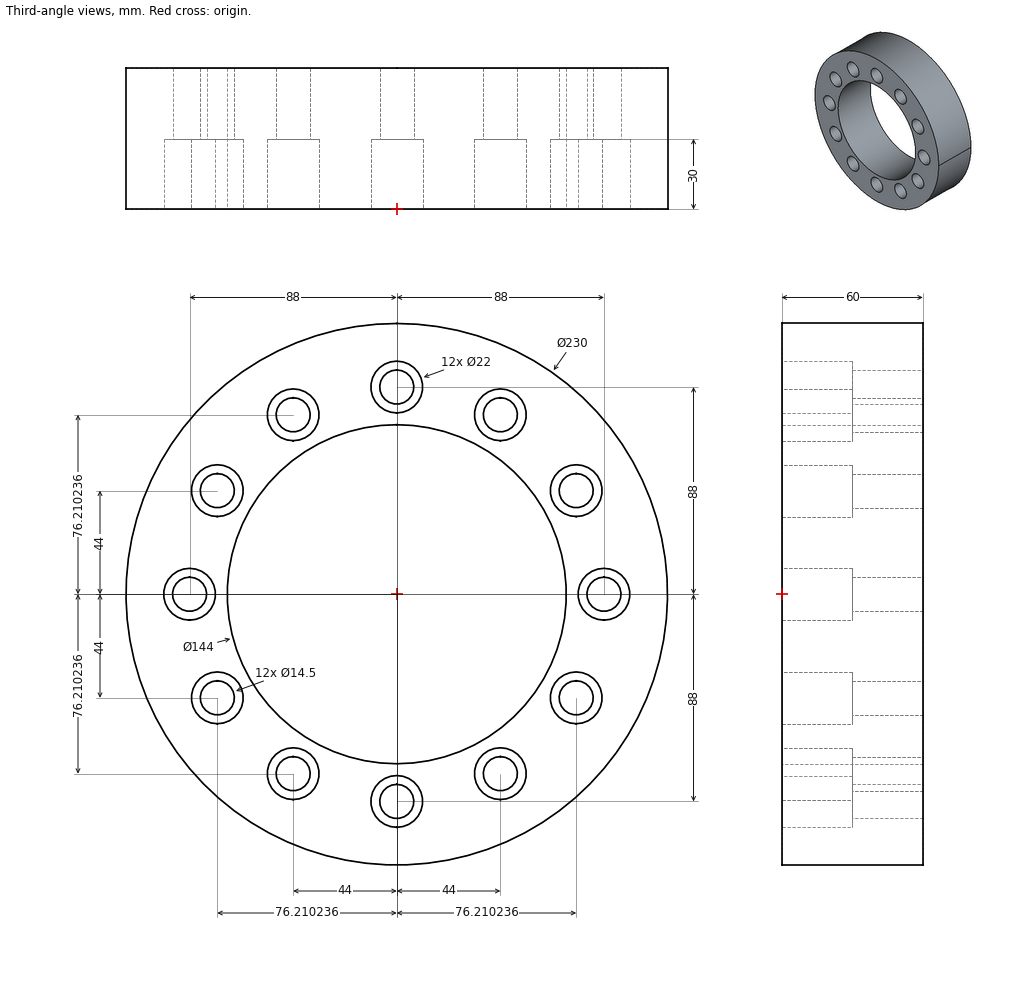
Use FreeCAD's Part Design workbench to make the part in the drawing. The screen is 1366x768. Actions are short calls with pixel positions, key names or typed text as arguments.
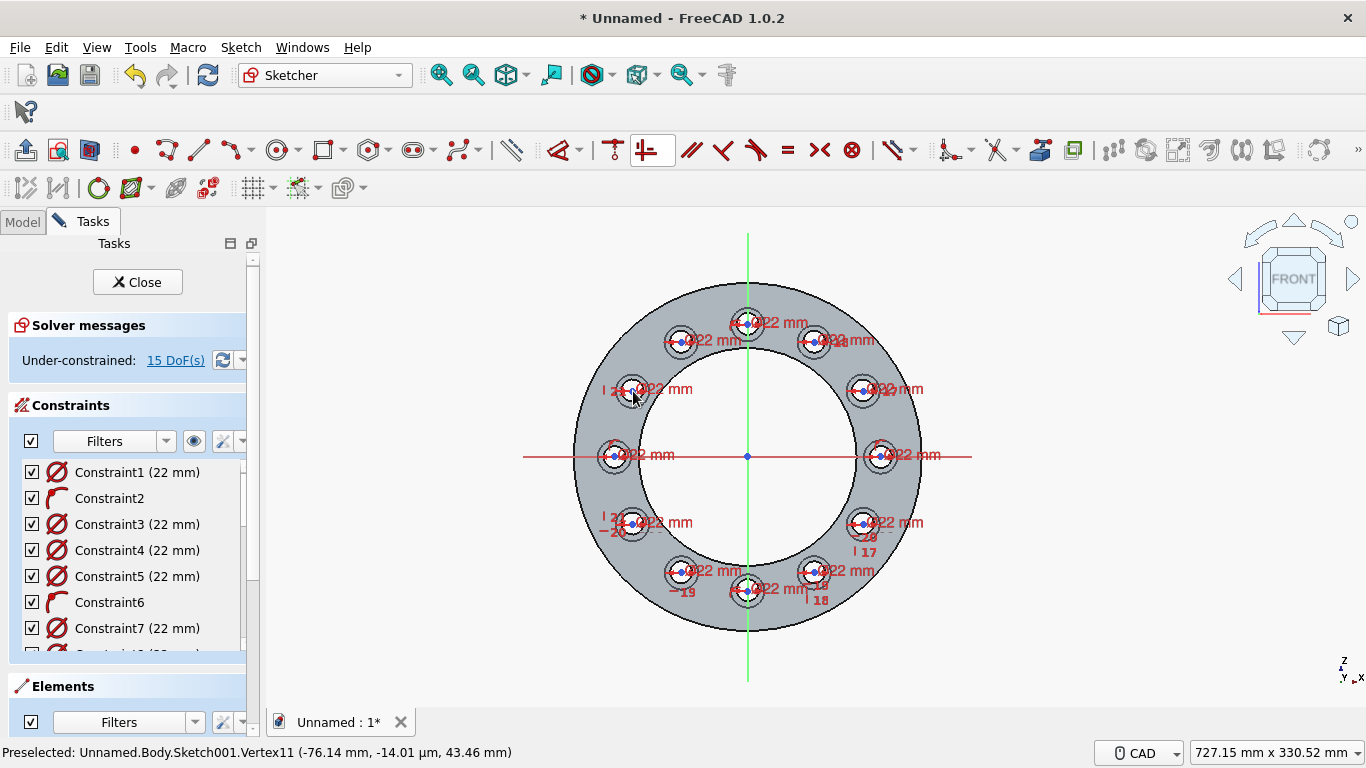
click(863, 391)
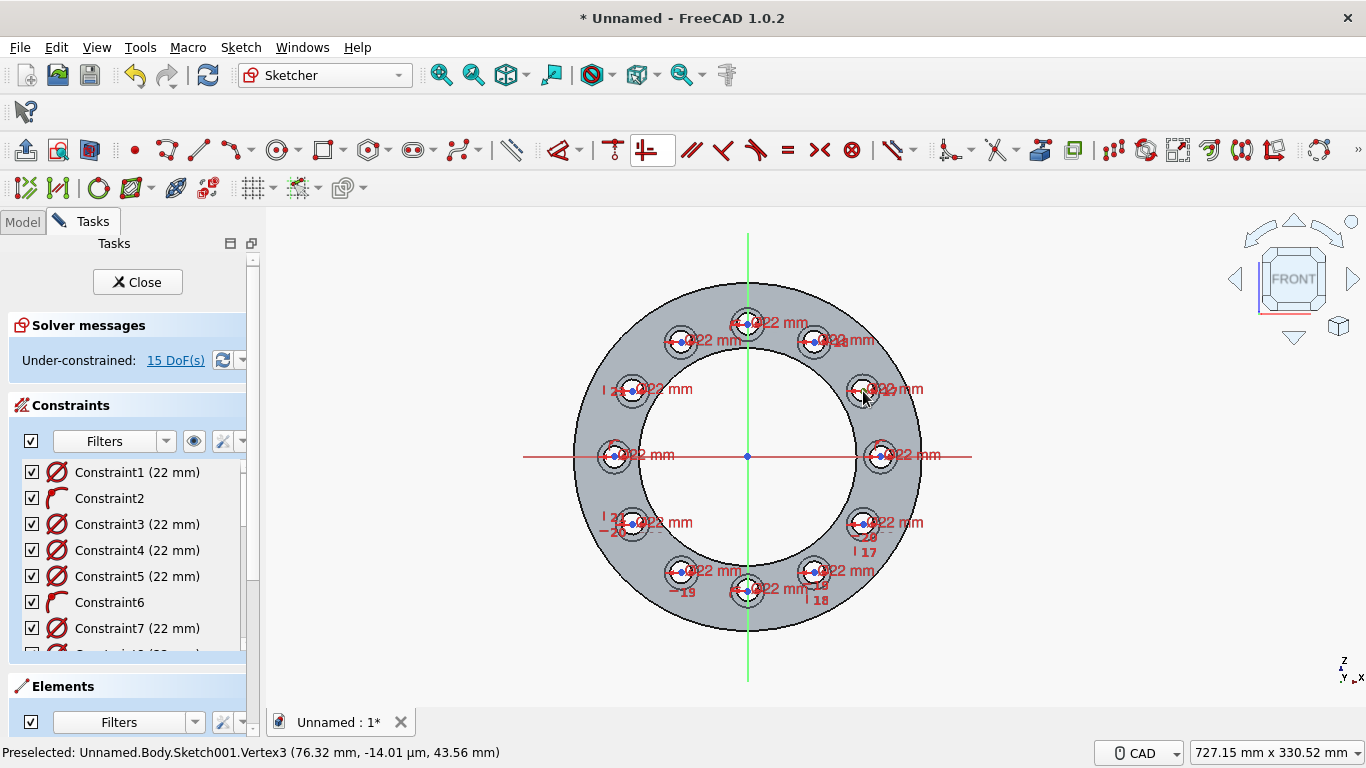
click(633, 391)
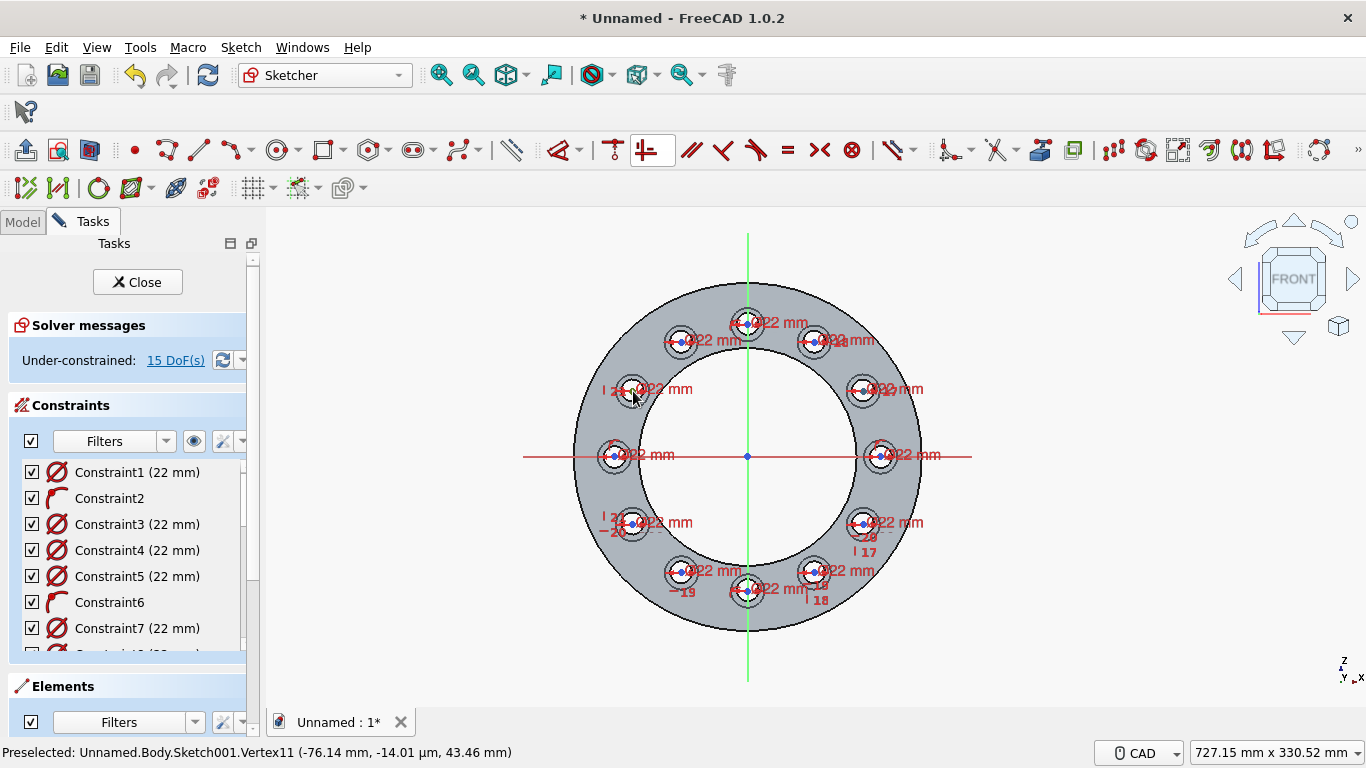
click(670, 150)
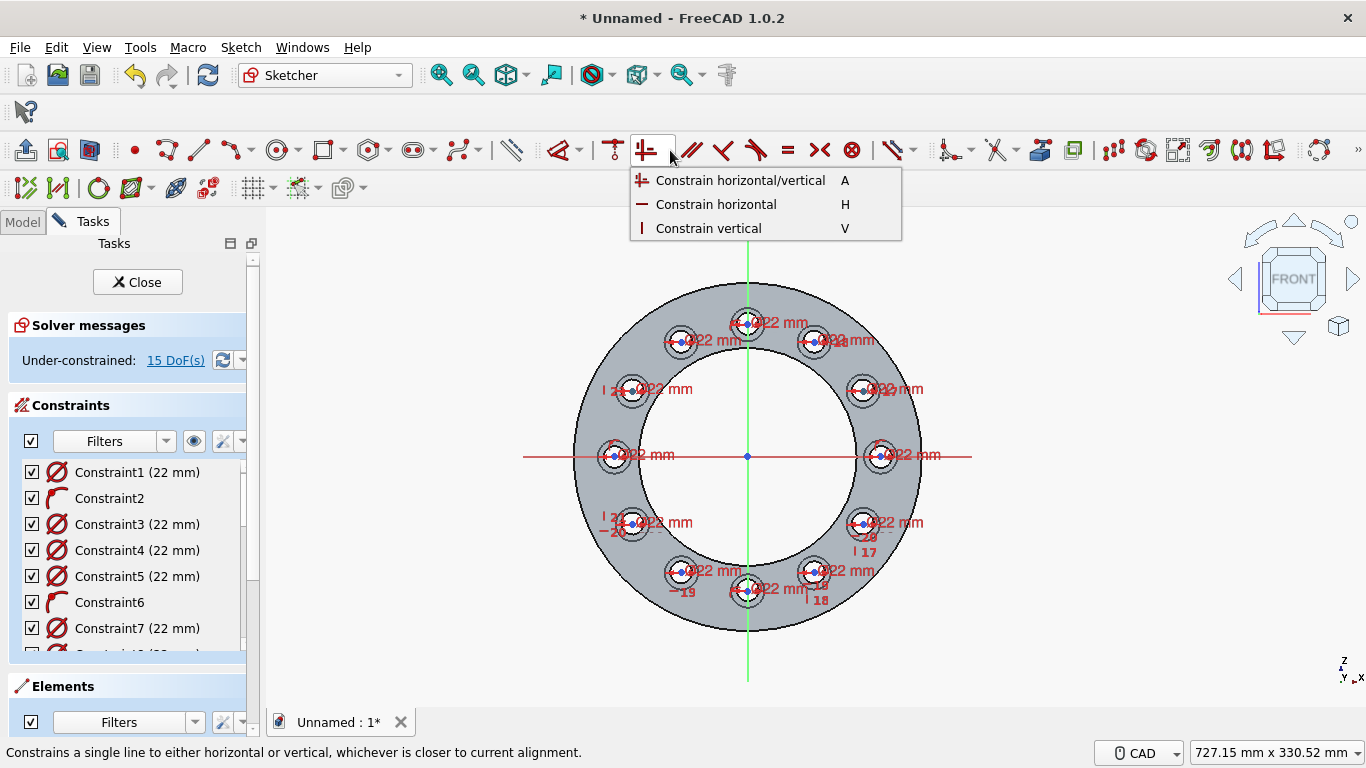
click(766, 204)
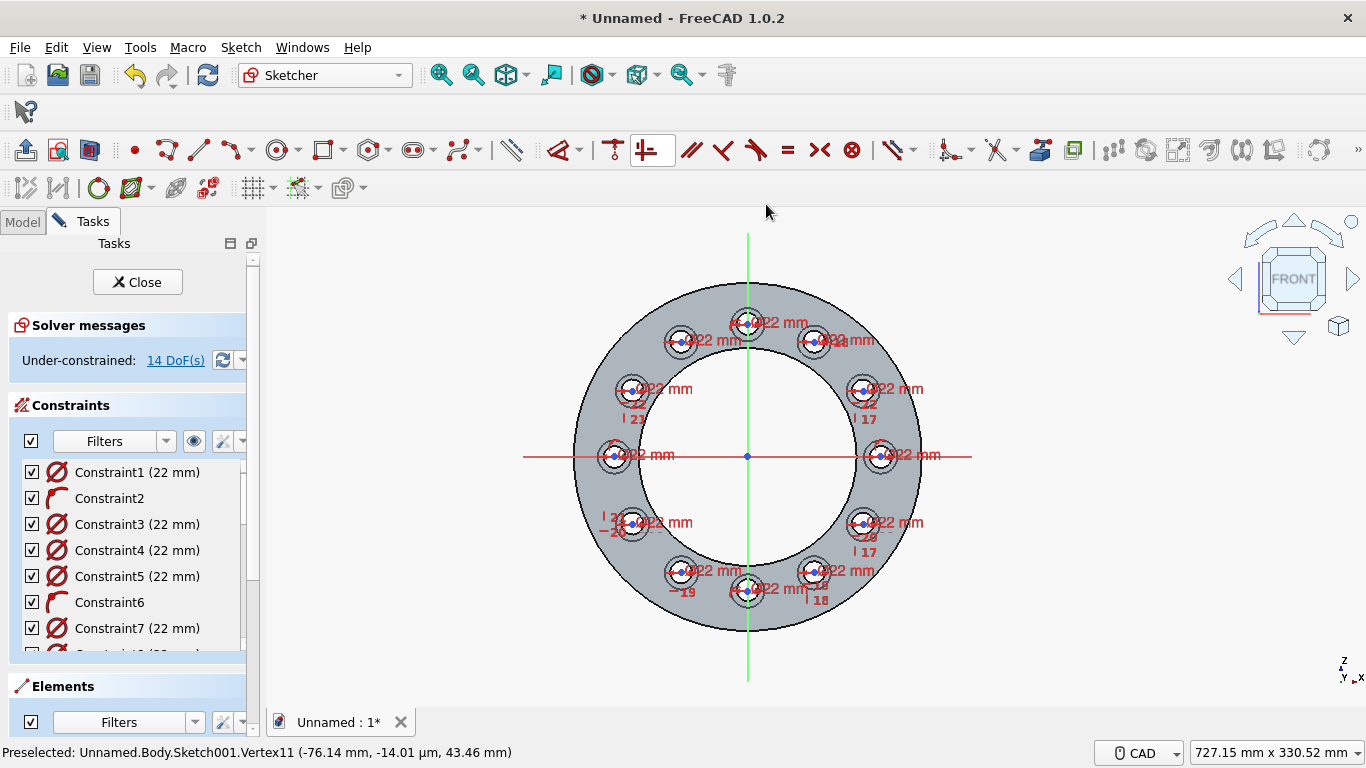
click(814, 342)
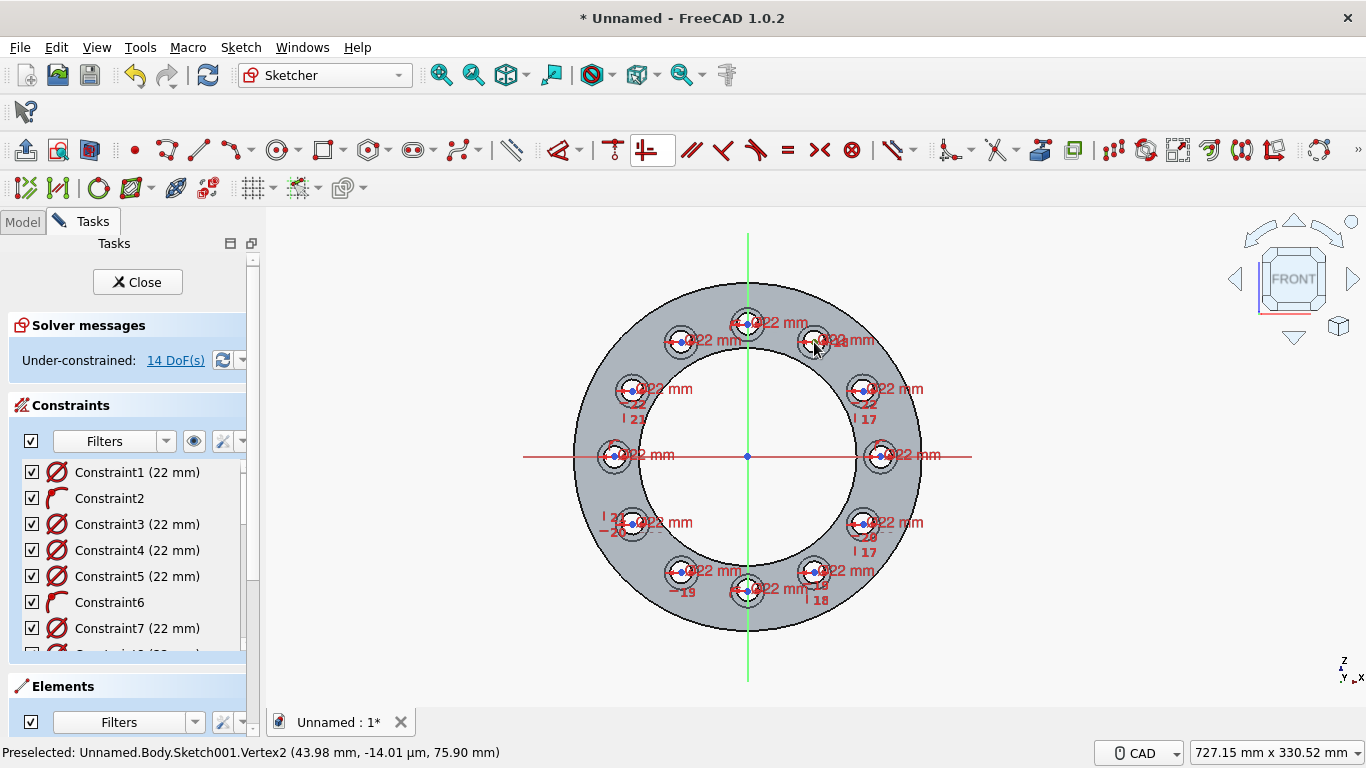
click(681, 342)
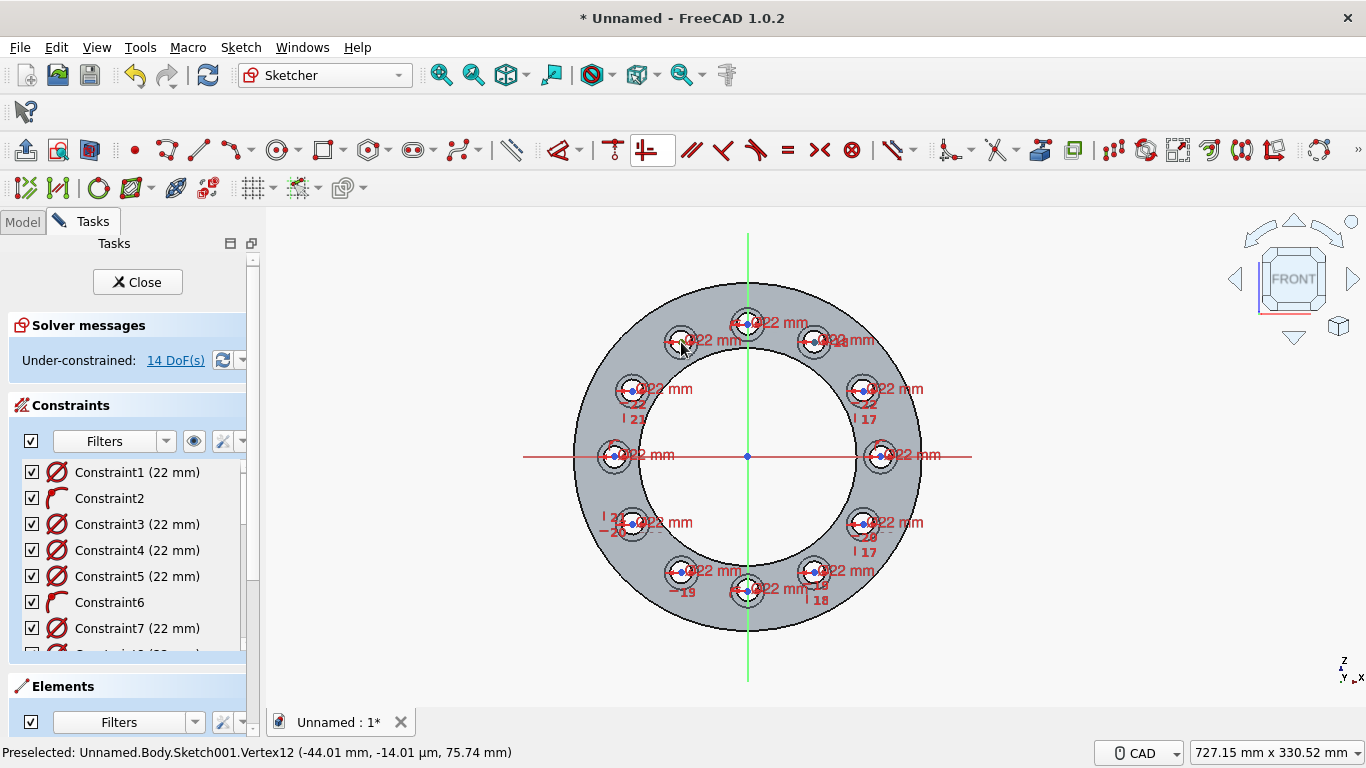
click(670, 150)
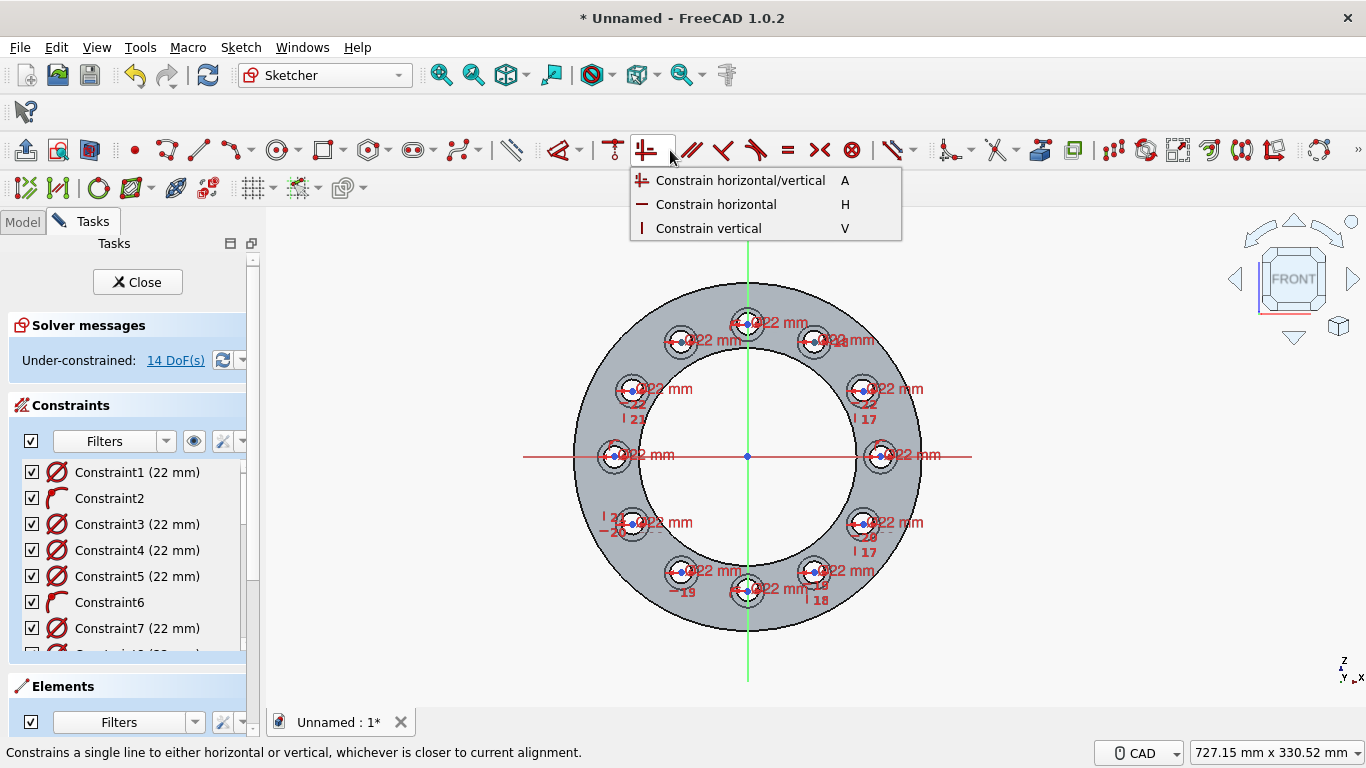
click(766, 204)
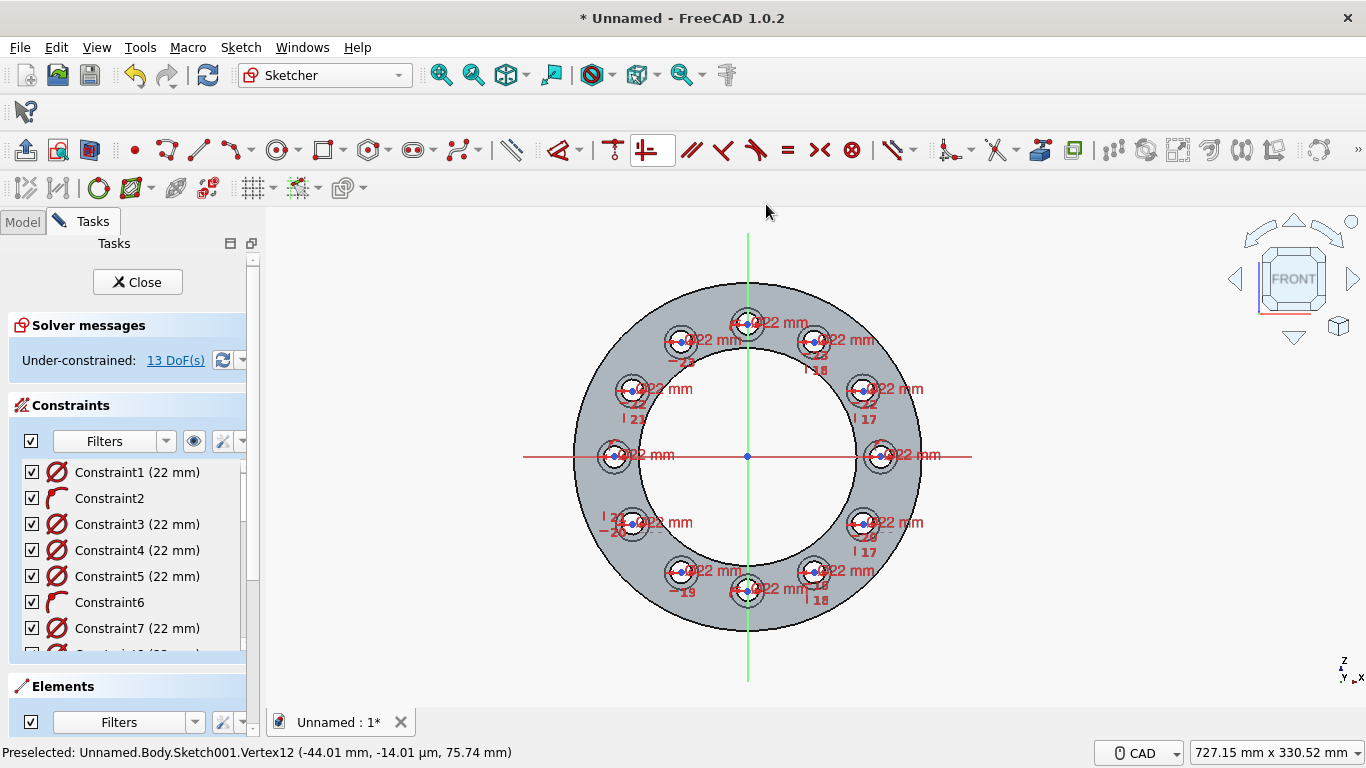
click(558, 150)